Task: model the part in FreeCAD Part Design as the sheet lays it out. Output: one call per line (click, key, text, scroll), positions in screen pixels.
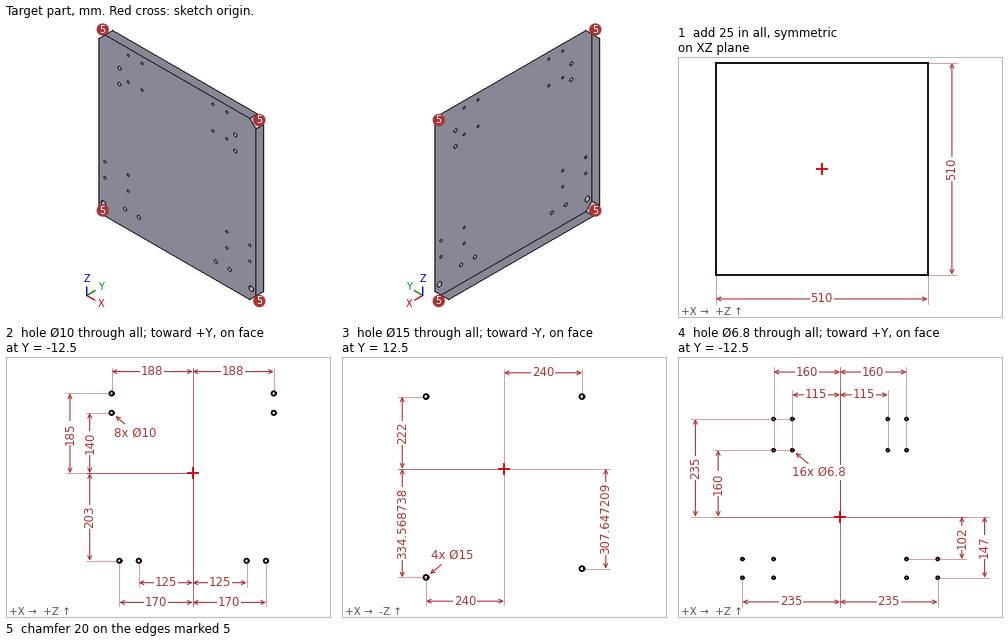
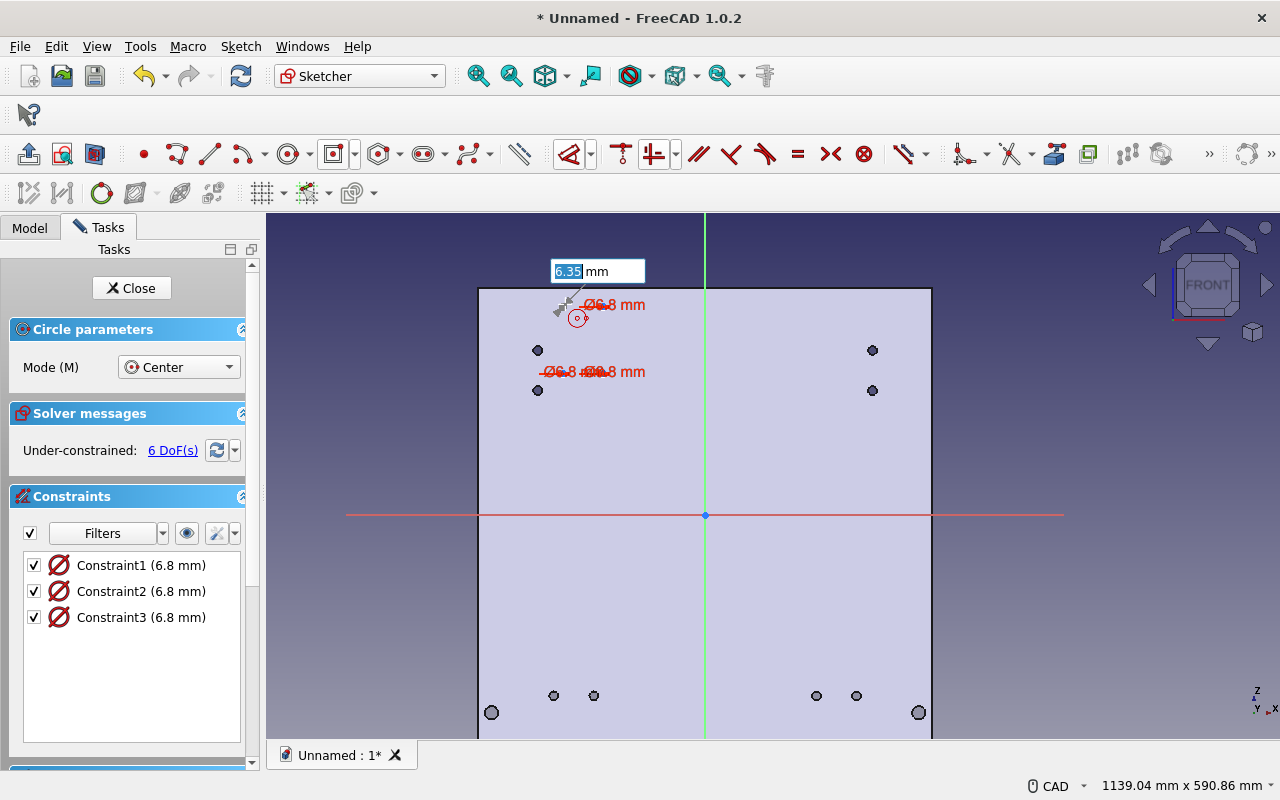
text(6.8)
key(Return)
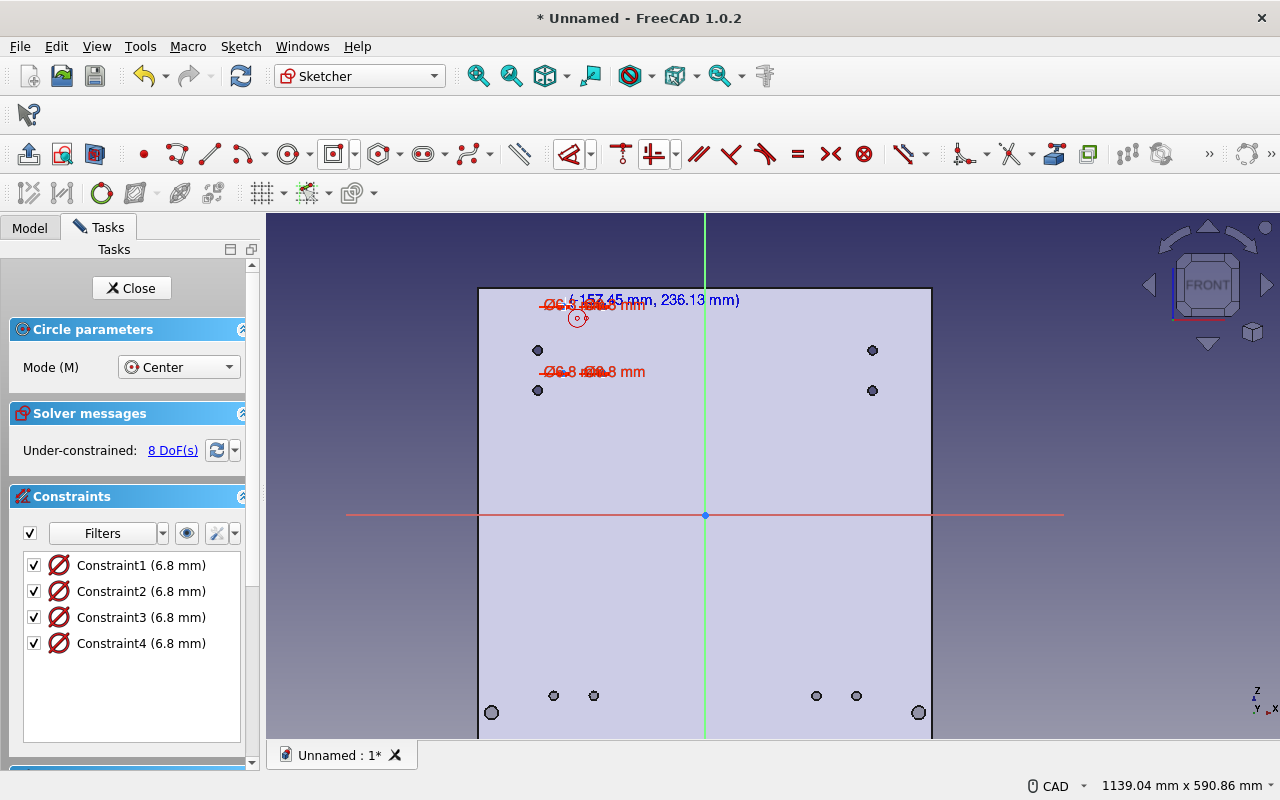
scroll(848, 373, up, 11)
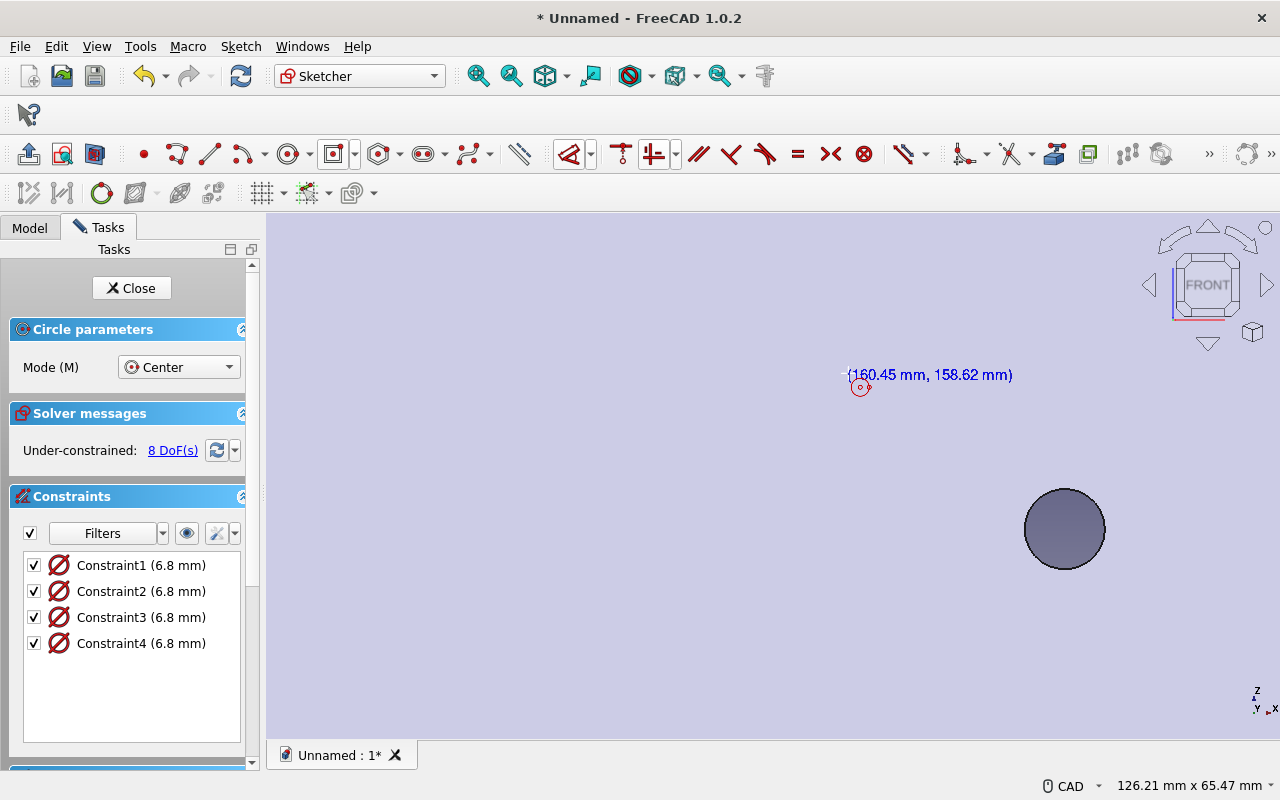
scroll(848, 373, down, 11)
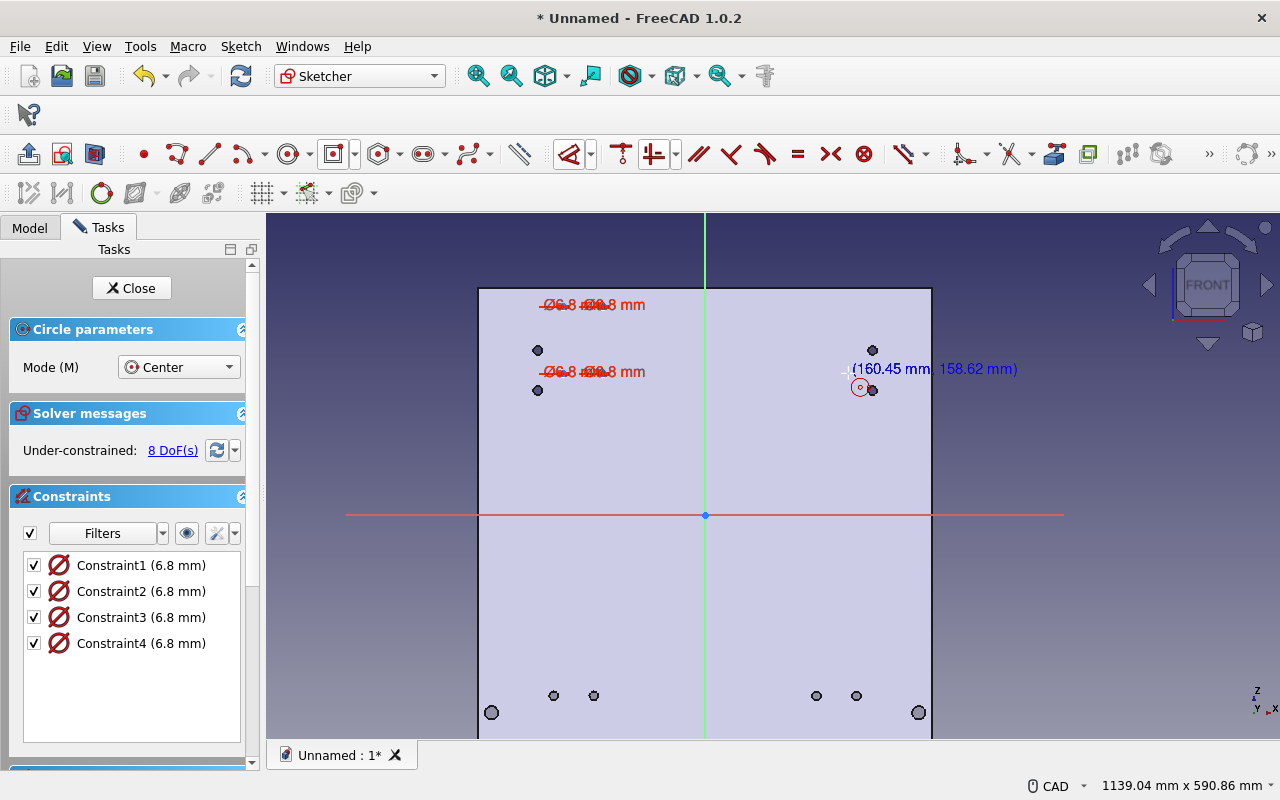
click(848, 373)
move(850, 371)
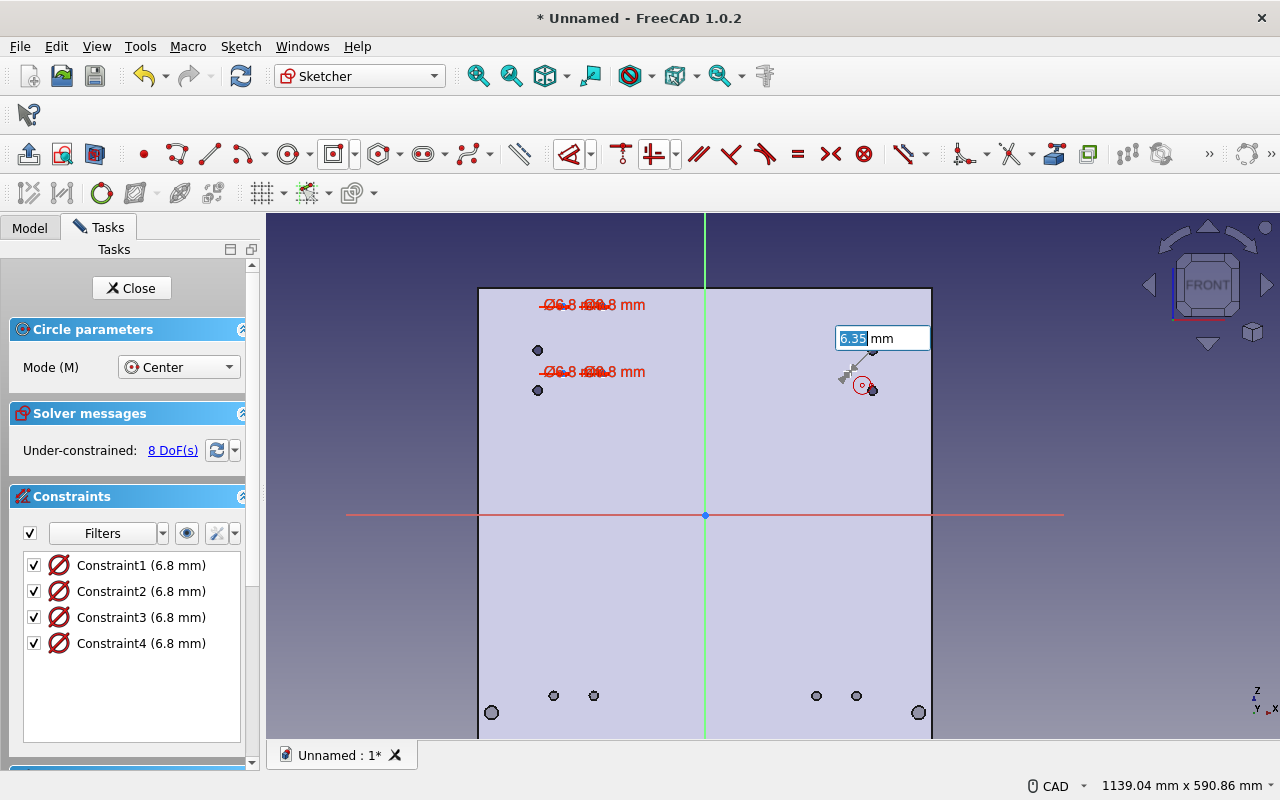
text(6.8)
key(Return)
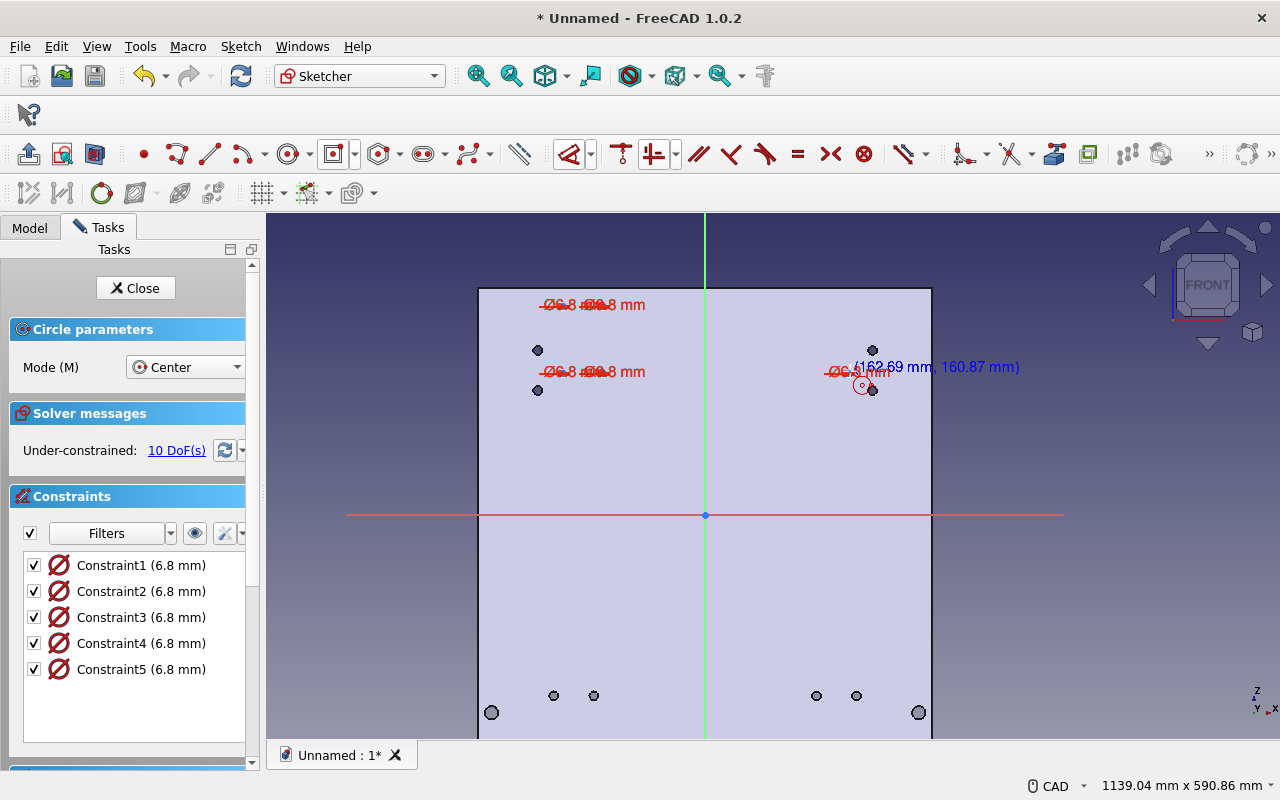
scroll(808, 373, up, 11)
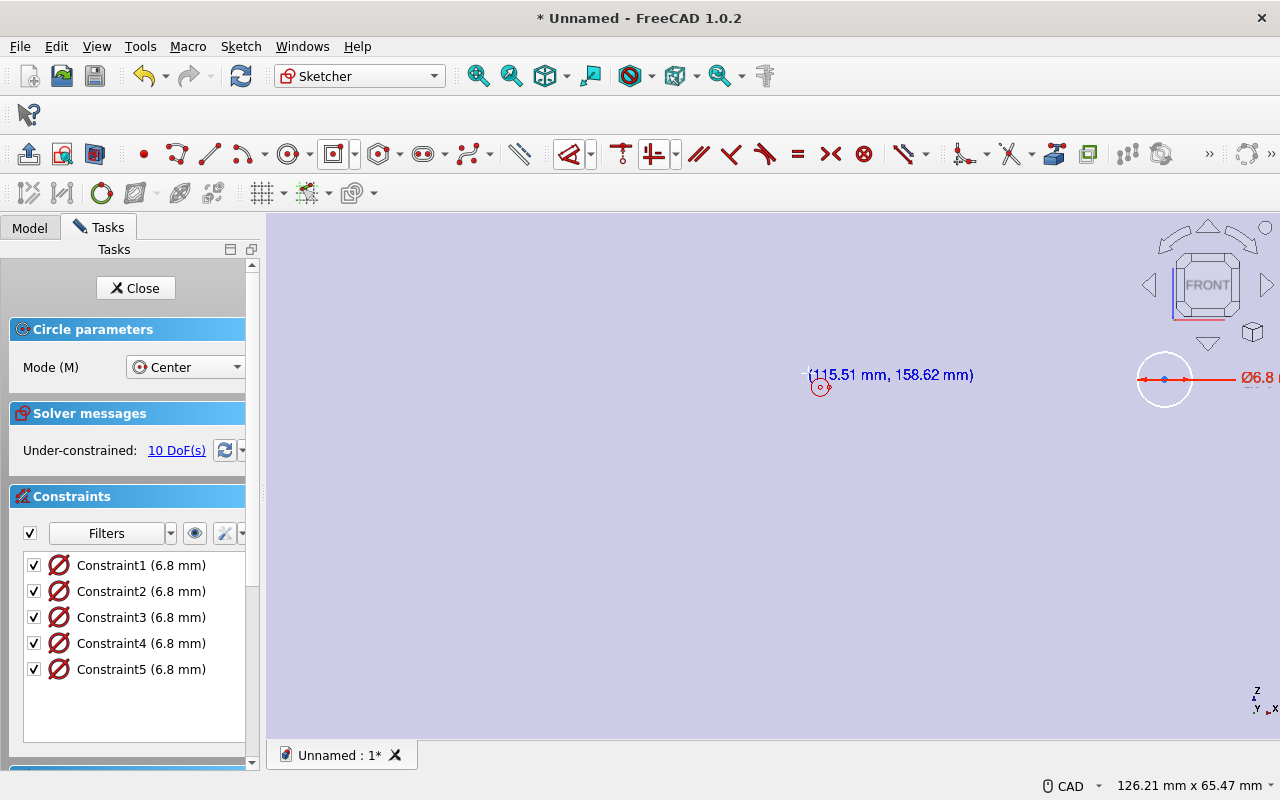
scroll(808, 373, down, 11)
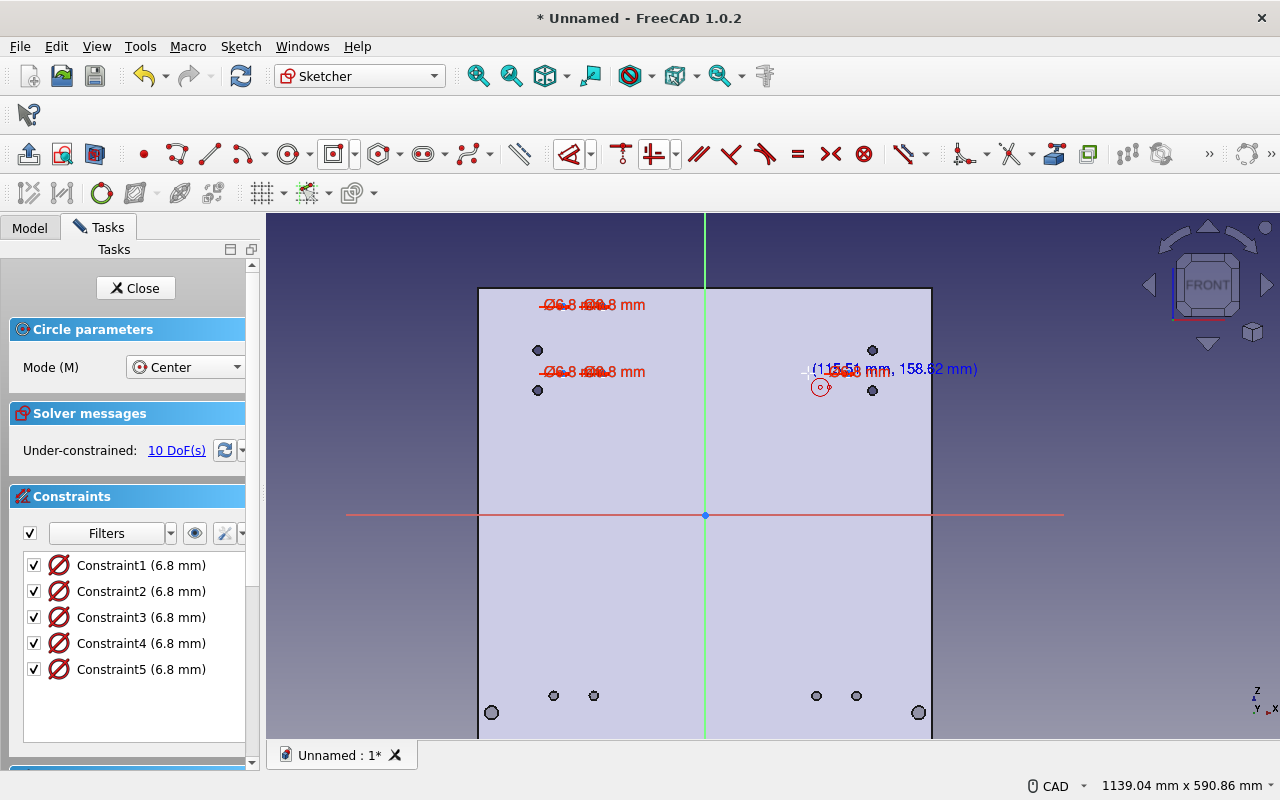
click(808, 373)
move(810, 371)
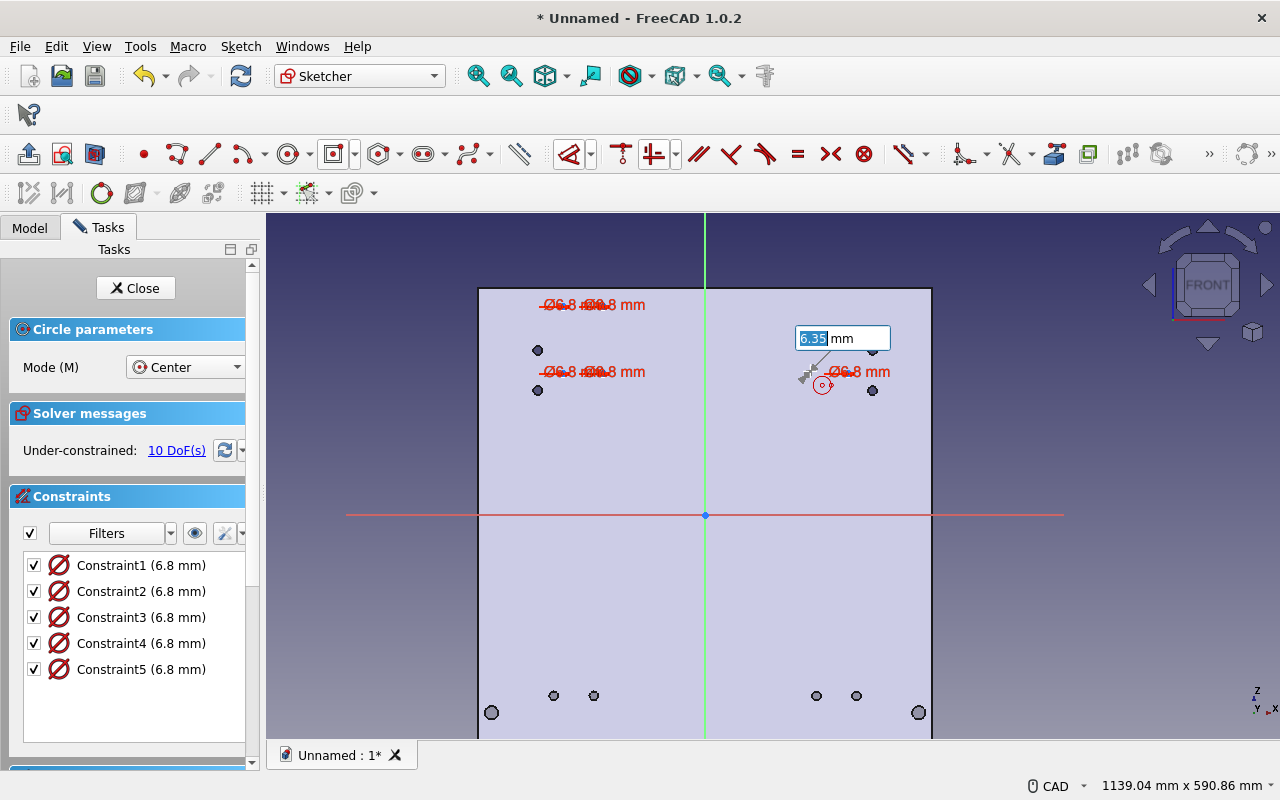
text(6.8)
key(Return)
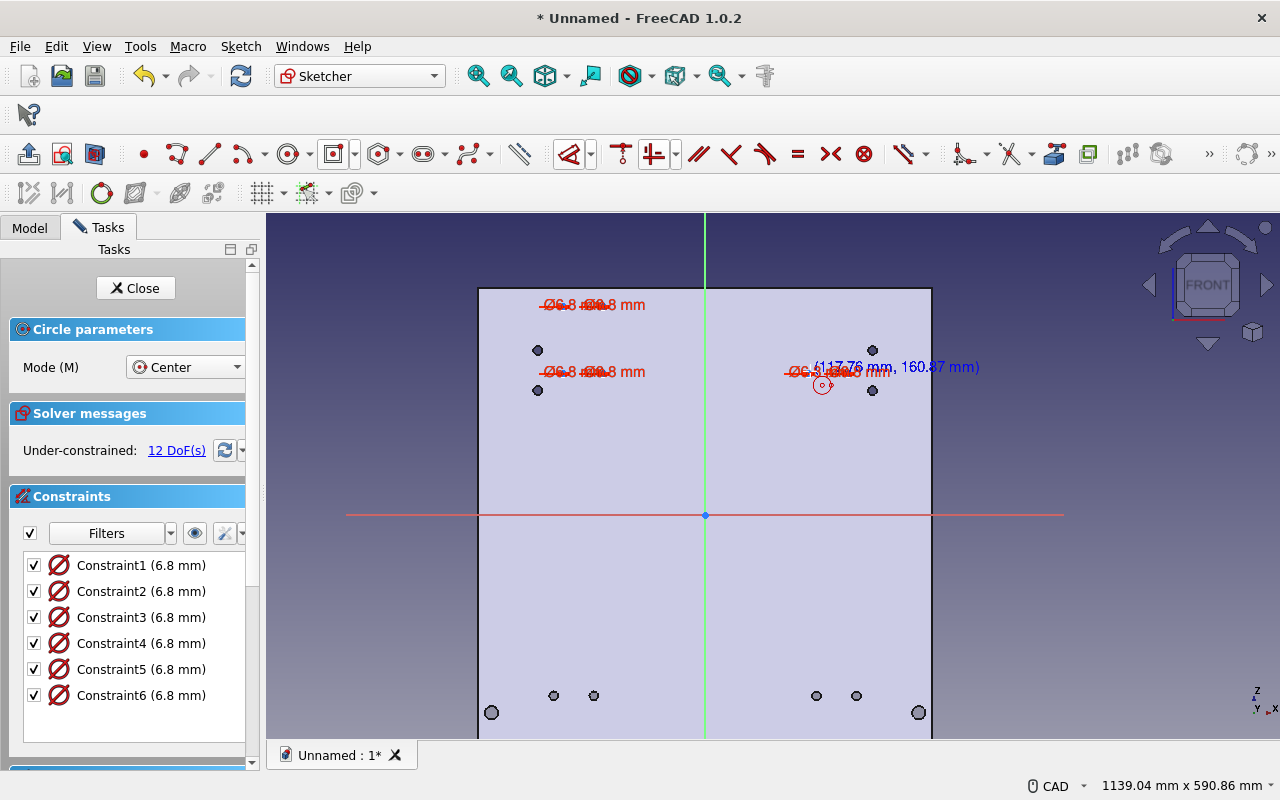
scroll(808, 306, up, 11)